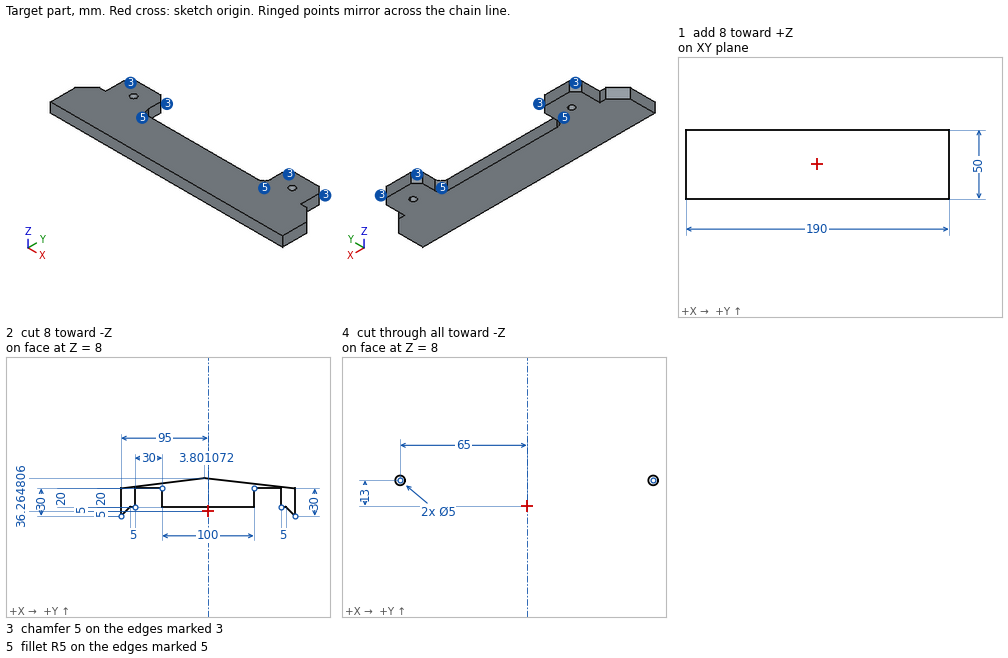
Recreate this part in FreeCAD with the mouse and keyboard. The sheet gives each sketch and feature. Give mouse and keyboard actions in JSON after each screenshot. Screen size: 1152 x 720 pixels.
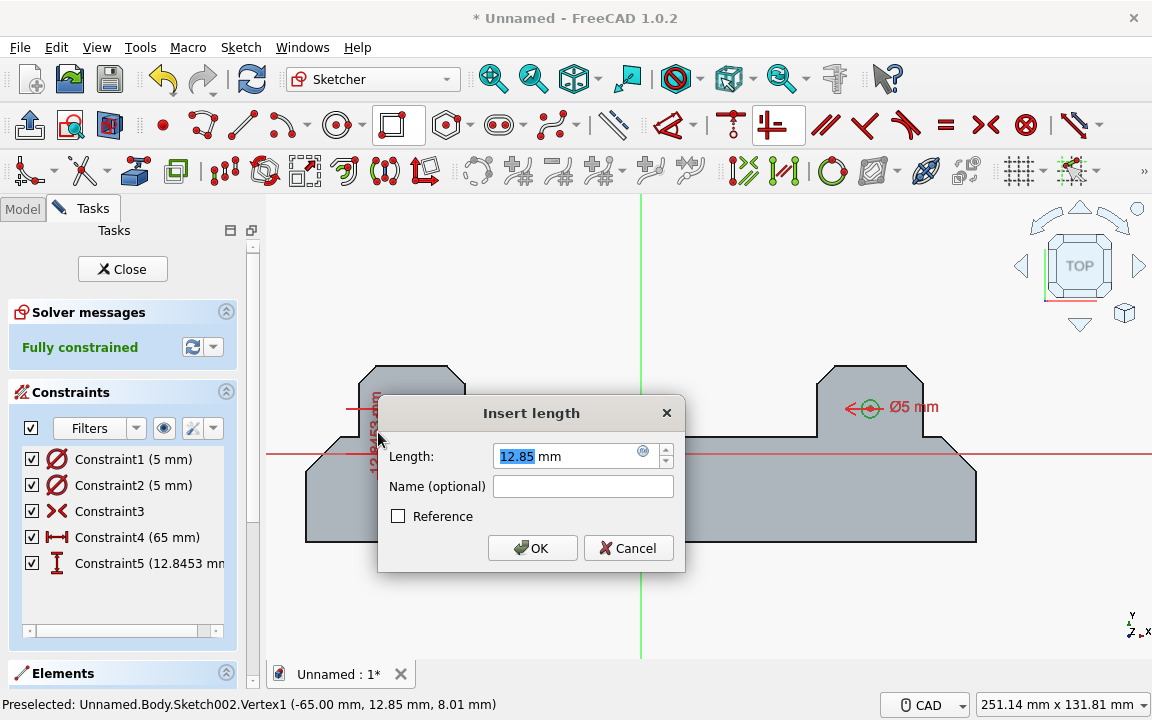
{"action": "type", "text": "13"}
{"action": "key", "text": "Return"}
{"action": "key", "text": "Escape"}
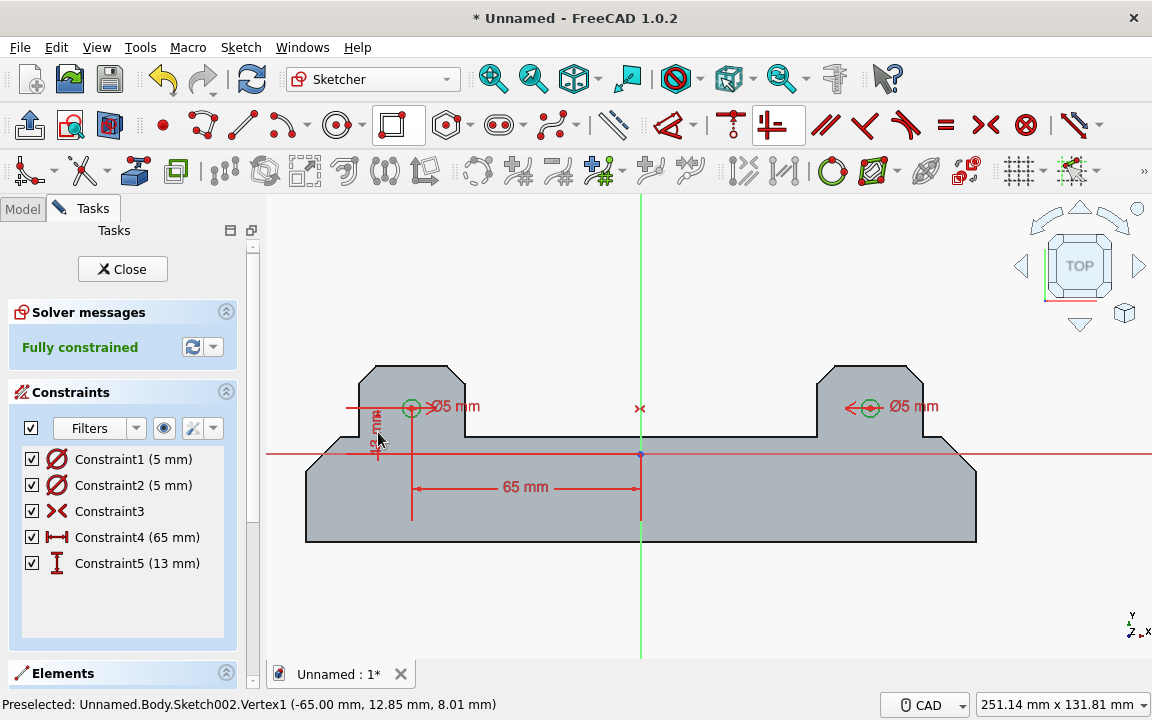
{"action": "left_click", "coordinate": [123, 269]}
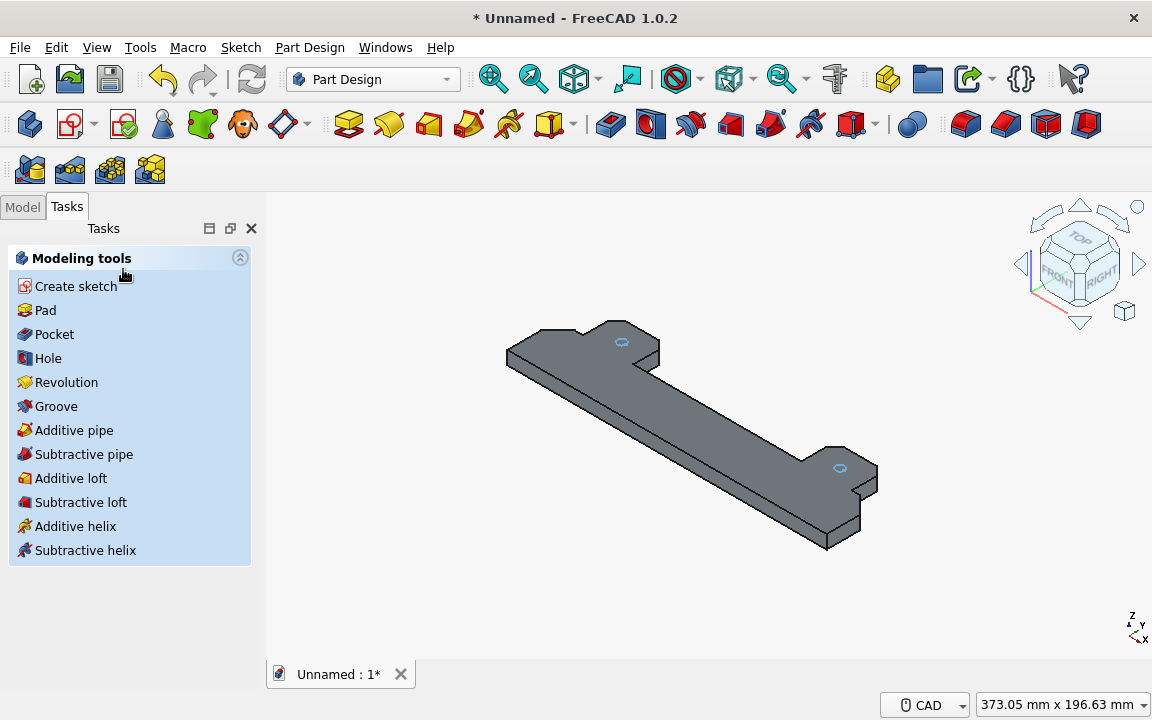
{"action": "left_click", "coordinate": [612, 124]}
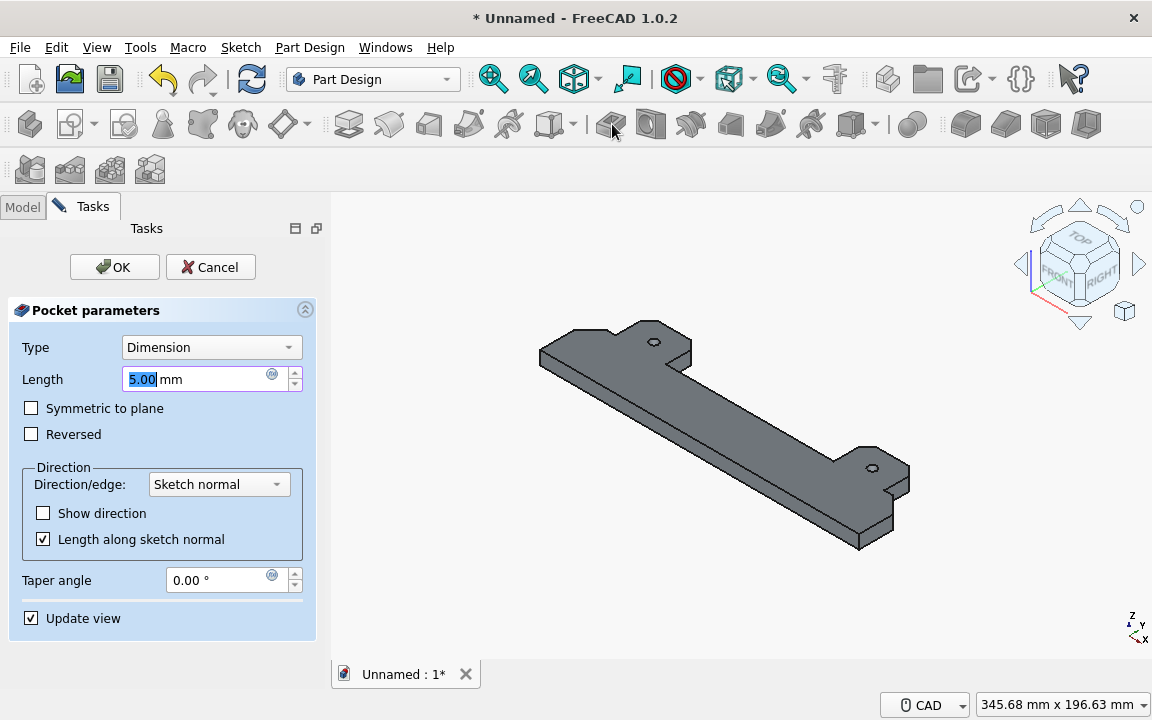
{"action": "left_click", "coordinate": [212, 348]}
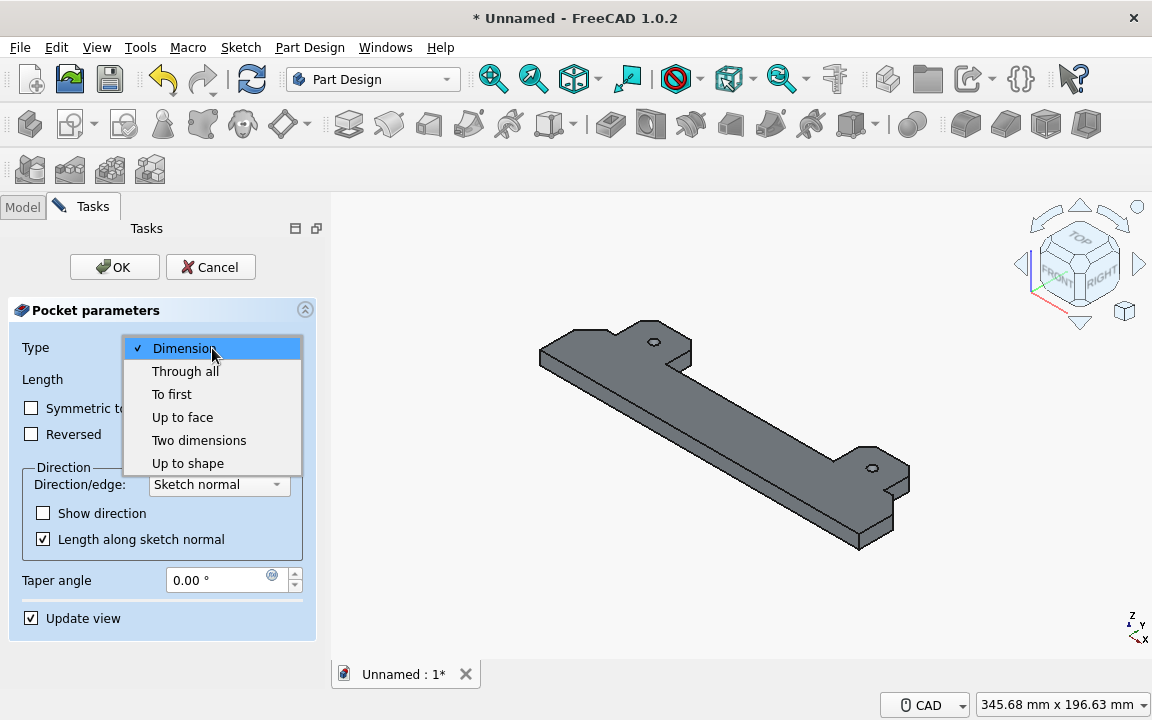
{"action": "left_click", "coordinate": [212, 372]}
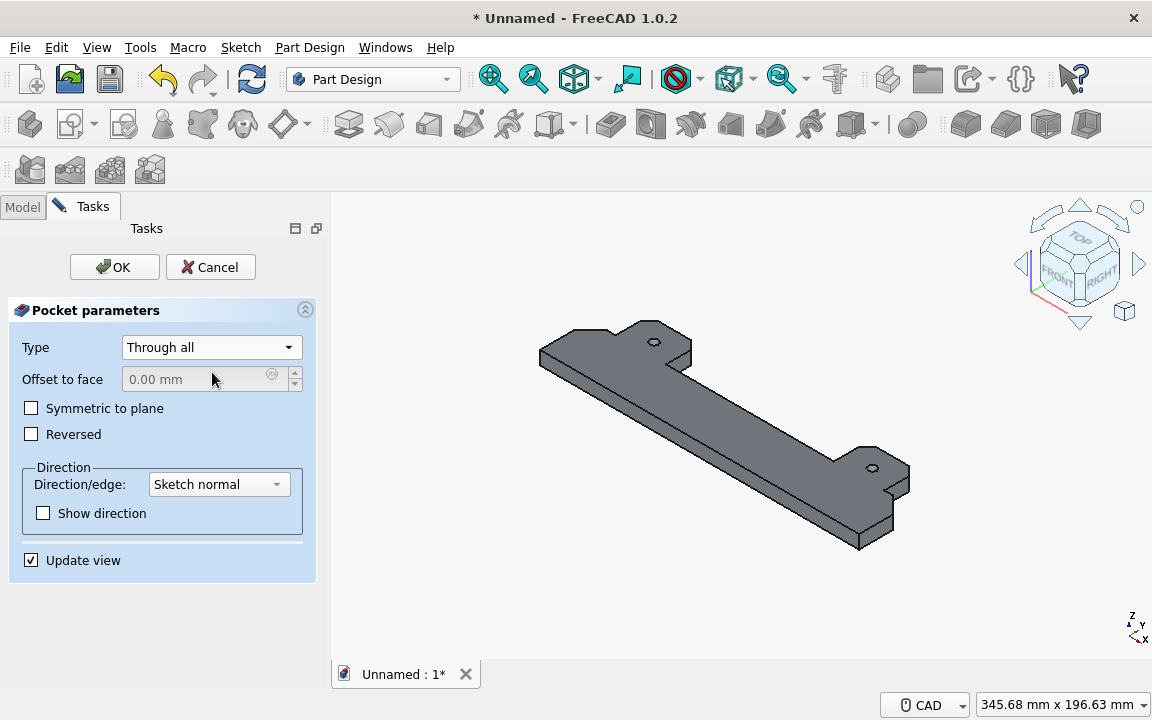
{"action": "left_click", "coordinate": [115, 267]}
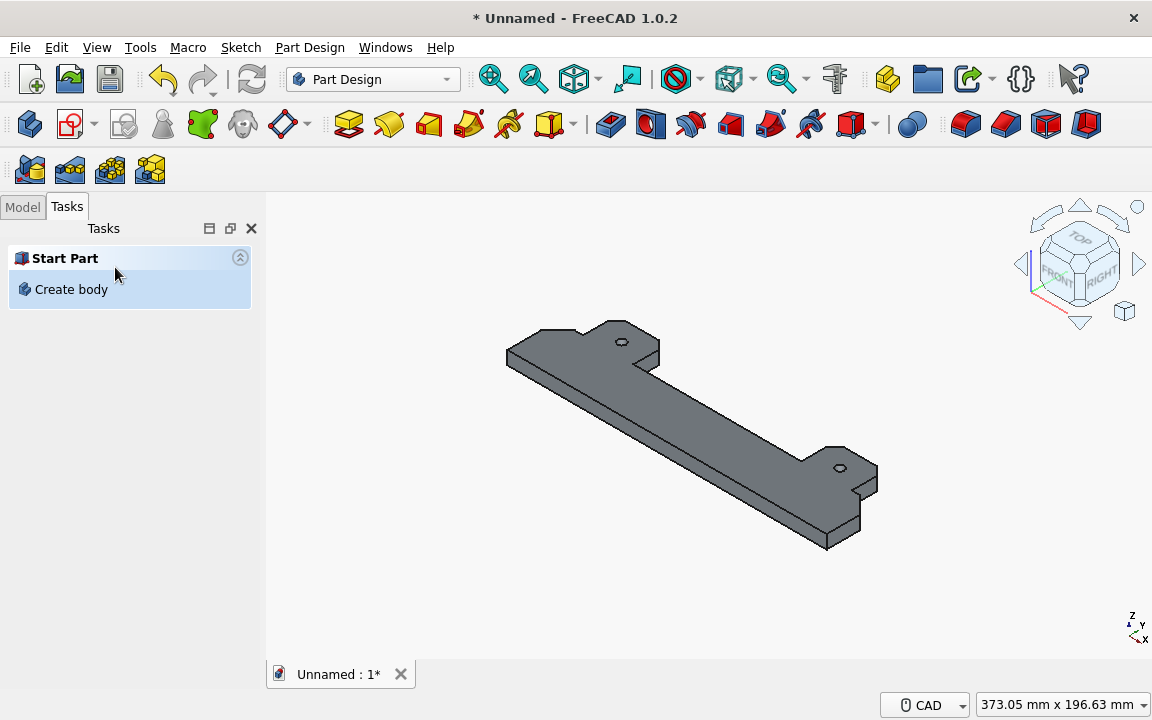
{"action": "scroll", "coordinate": [801, 468], "scroll_direction": "up", "scroll_amount": 4}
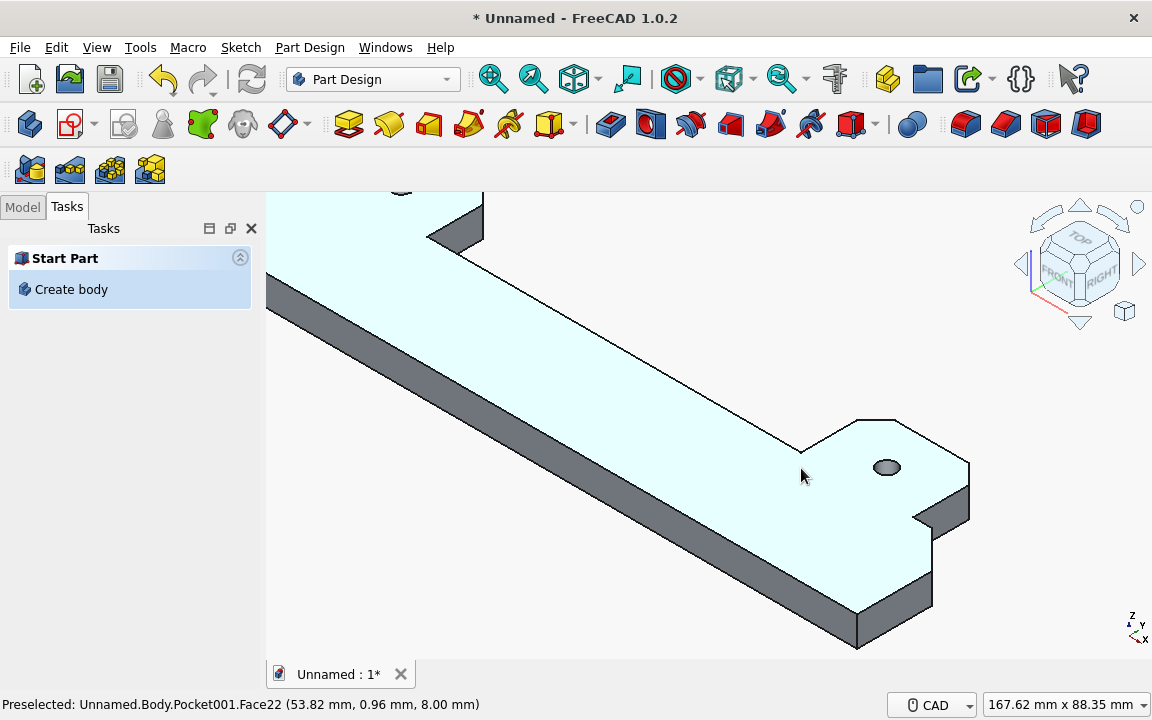
{"action": "left_click", "coordinate": [494, 80]}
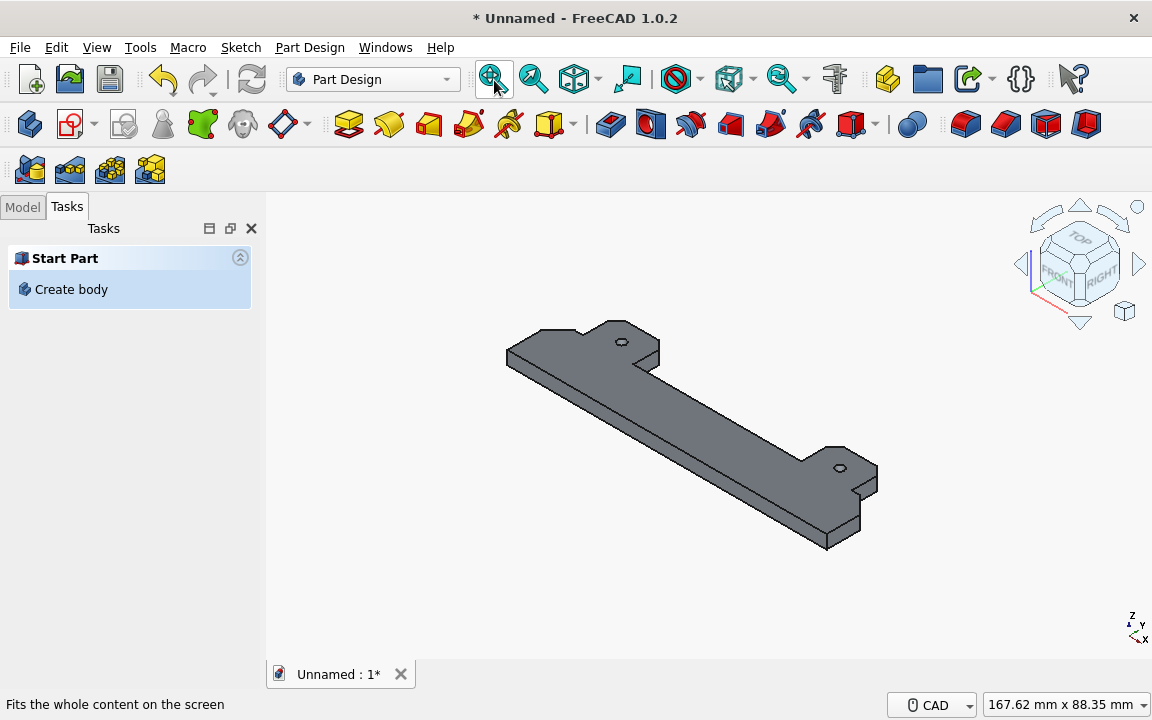
{"action": "key", "text": "2"}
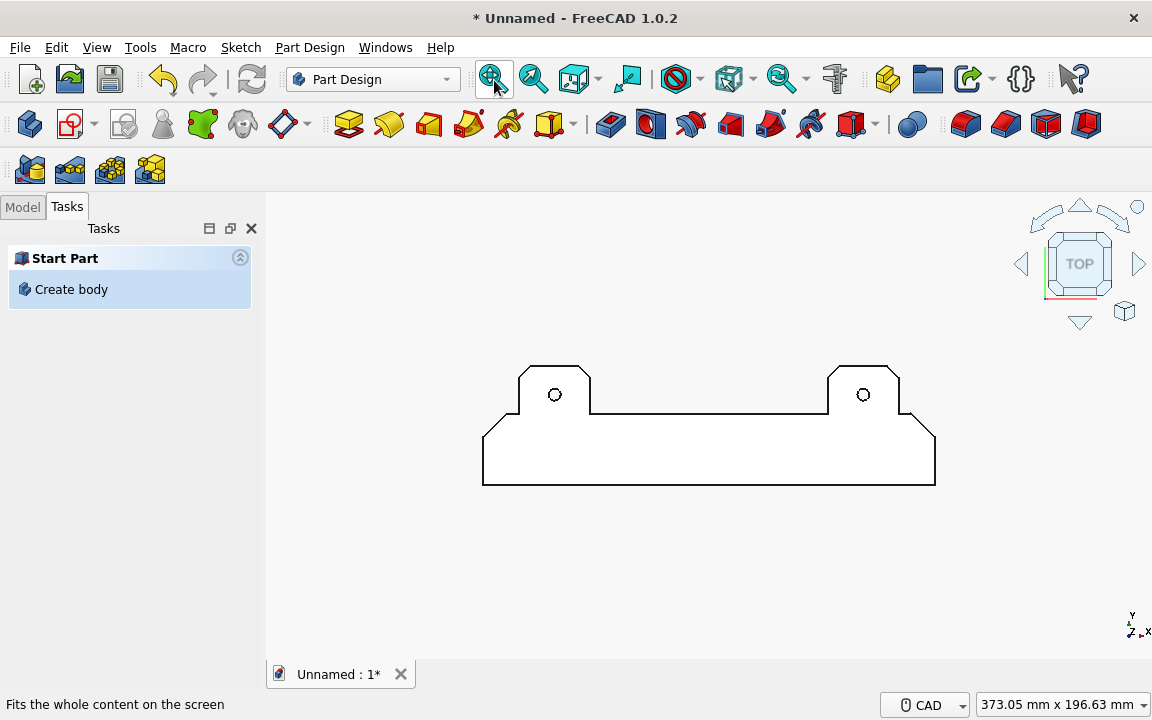
{"action": "scroll", "coordinate": [828, 413], "scroll_direction": "up", "scroll_amount": 4}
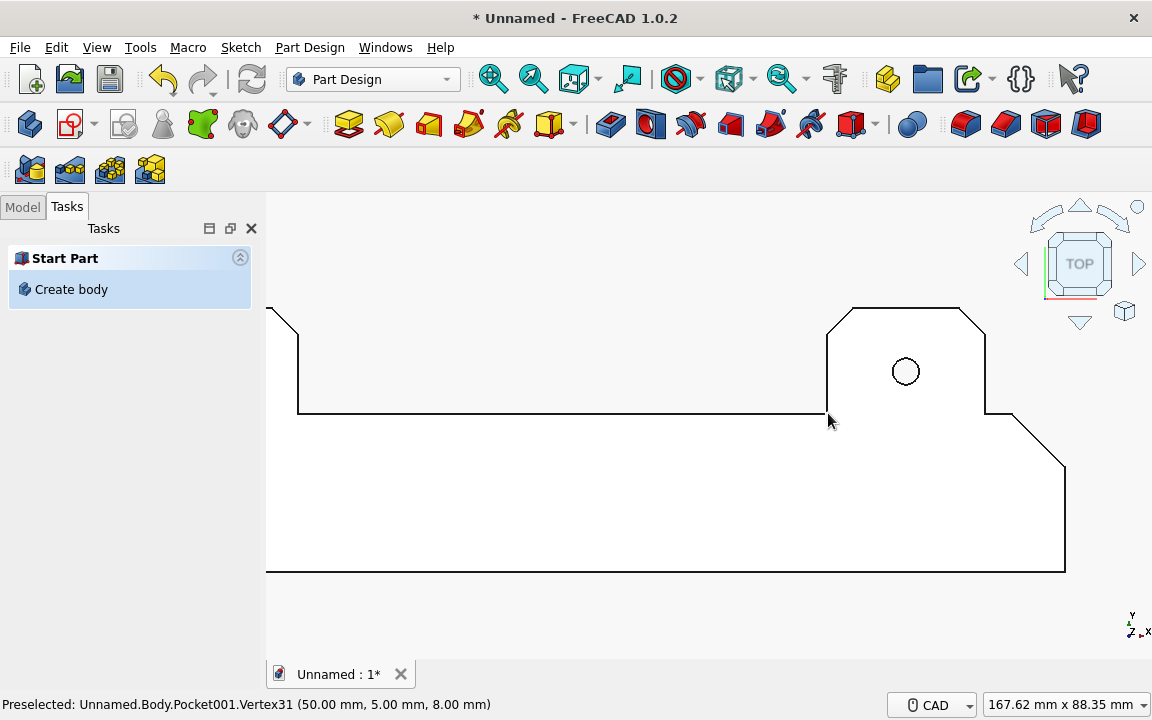
{"action": "key", "text": "v f"}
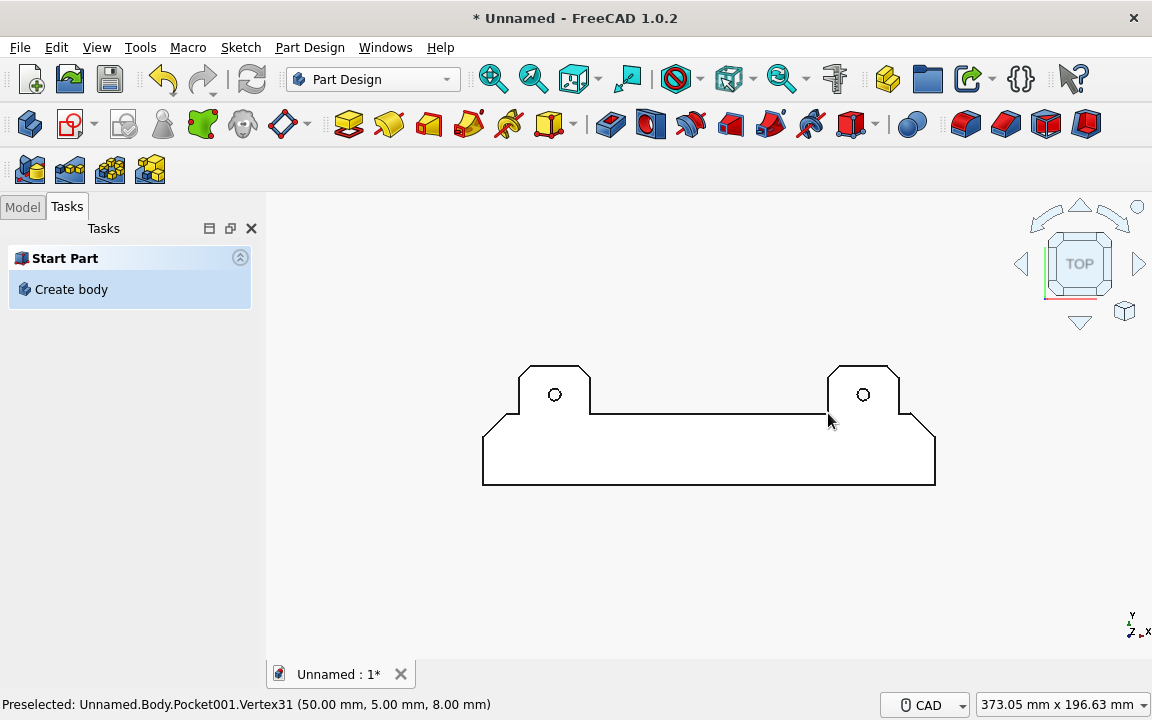
{"action": "key", "text": "0"}